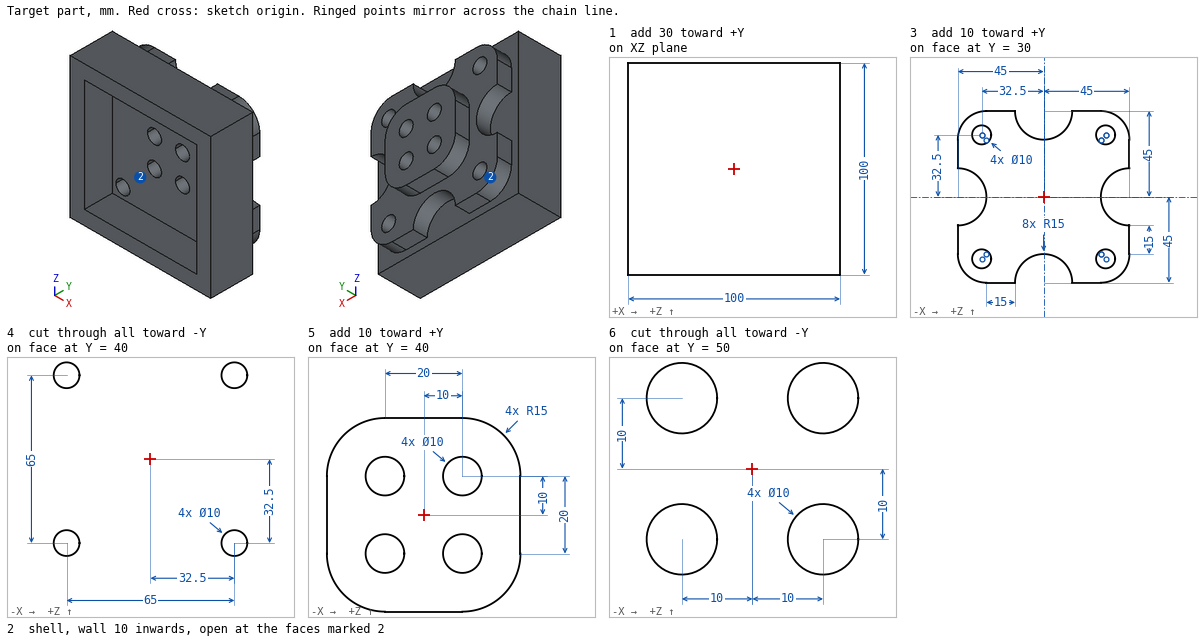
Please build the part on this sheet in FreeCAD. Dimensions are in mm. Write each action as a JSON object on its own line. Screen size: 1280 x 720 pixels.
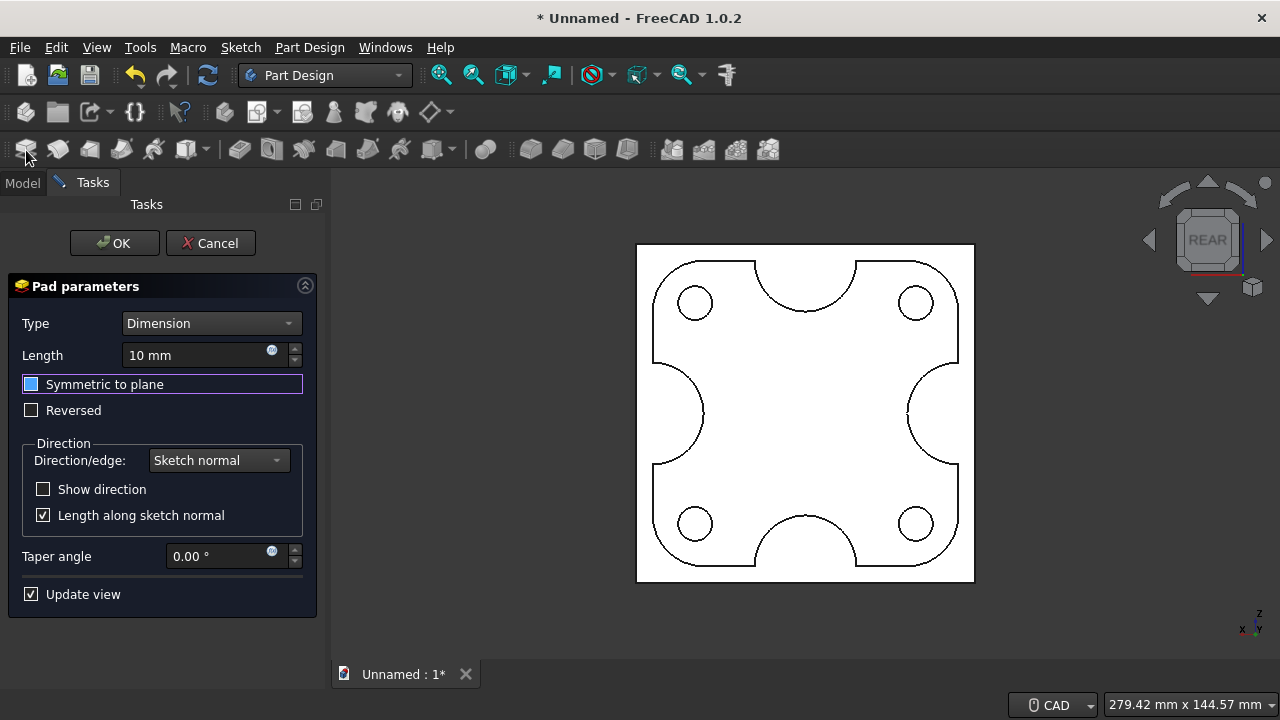
{"action": "left_click", "coordinate": [115, 243]}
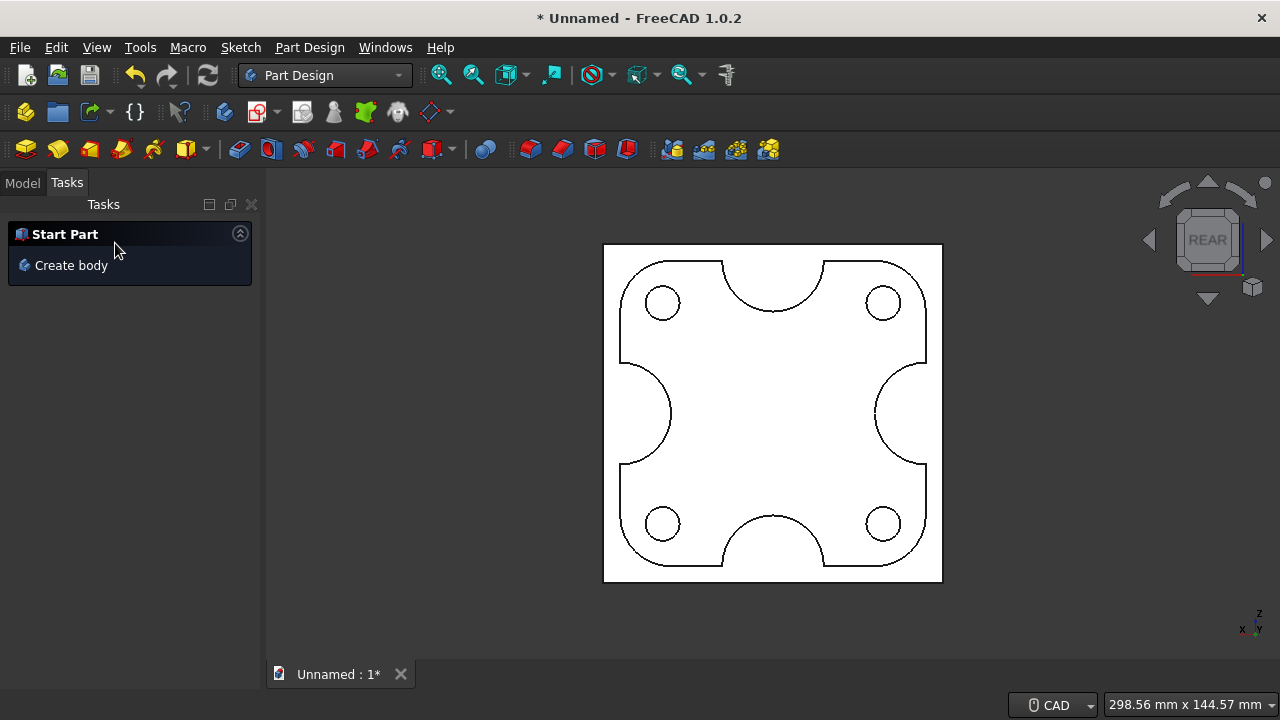
{"action": "left_click", "coordinate": [773, 412]}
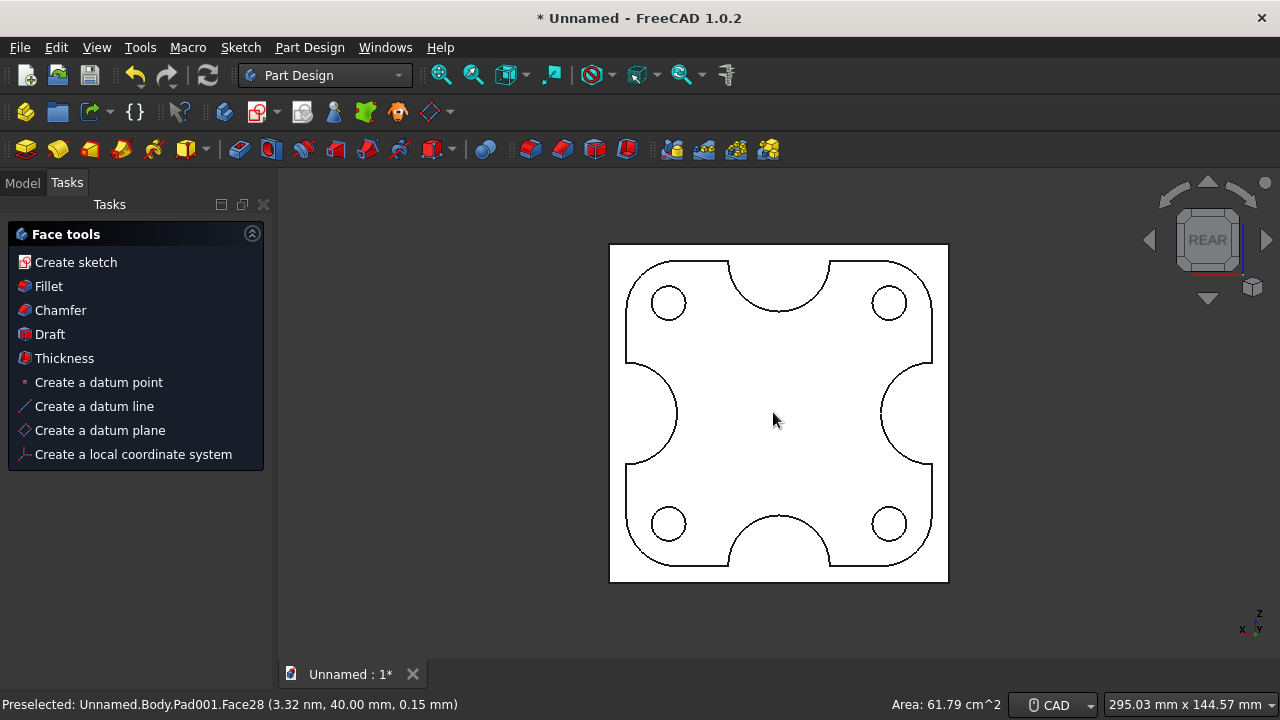
{"action": "left_click", "coordinate": [258, 112]}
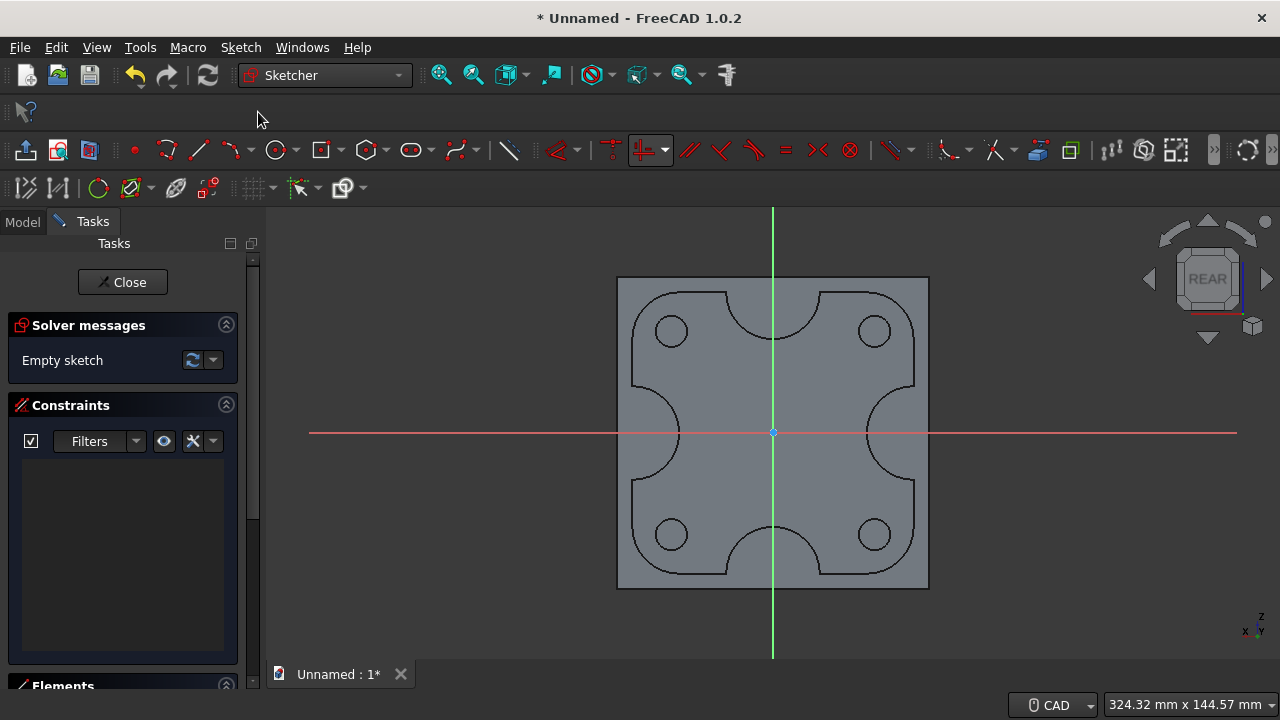
{"action": "left_click", "coordinate": [276, 150]}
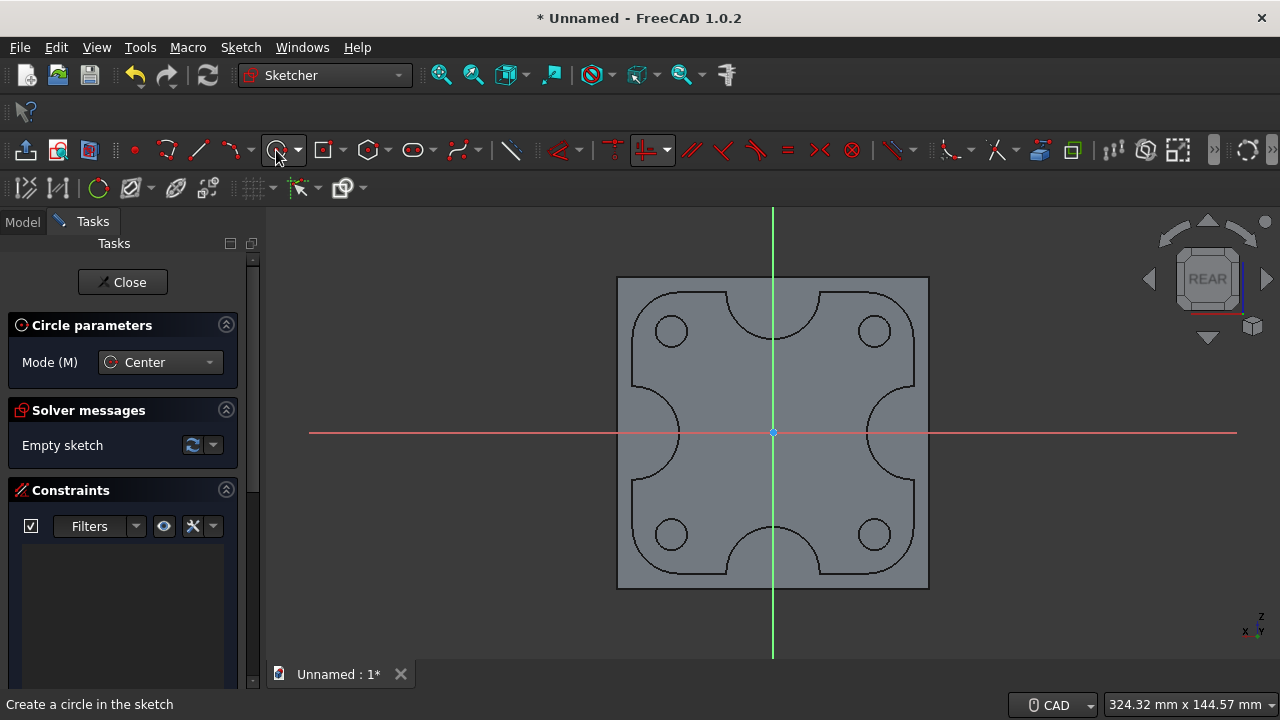
{"action": "scroll", "coordinate": [875, 535], "scroll_direction": "up", "scroll_amount": 2}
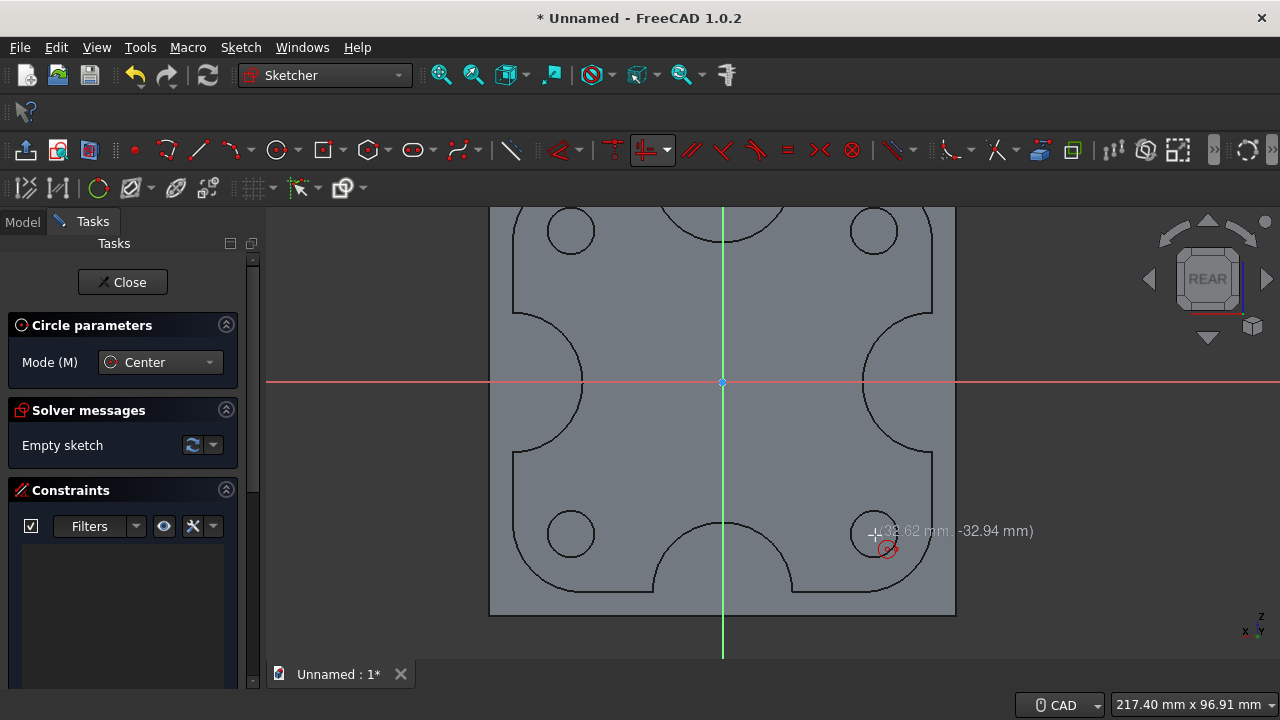
{"action": "left_click", "coordinate": [874, 534]}
{"action": "left_click", "coordinate": [891, 518]}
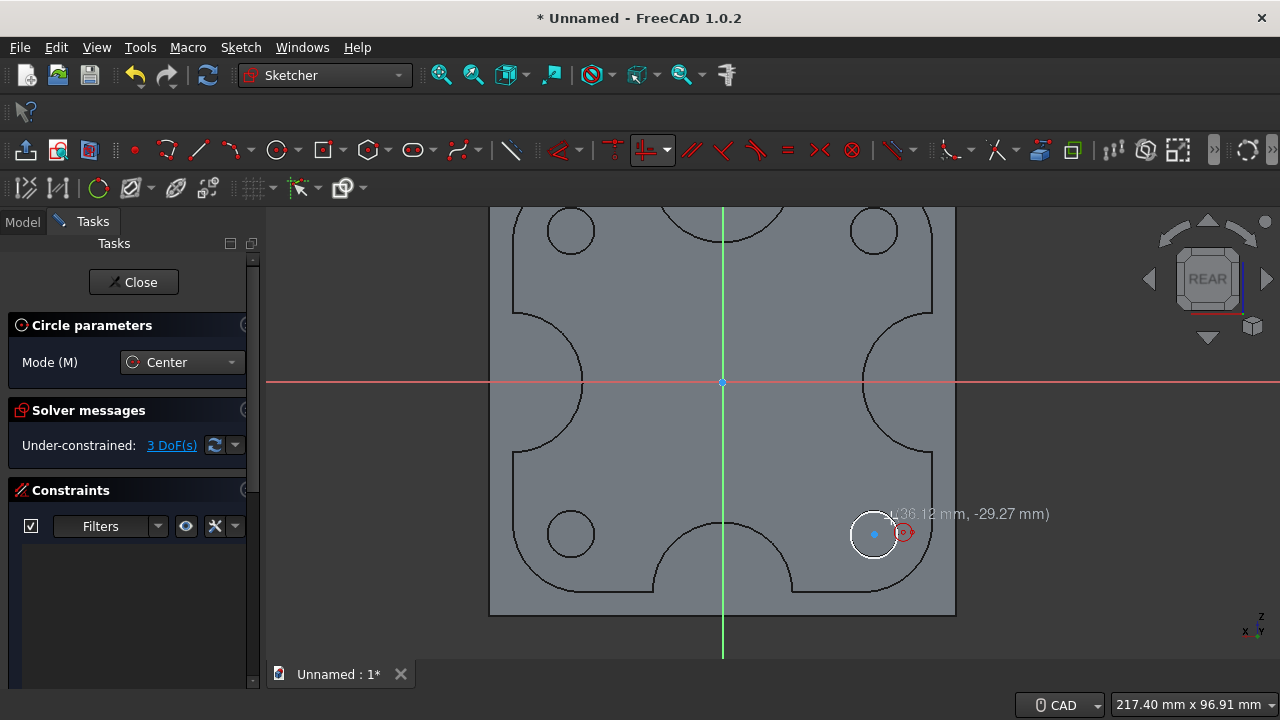
{"action": "left_click", "coordinate": [571, 534]}
{"action": "left_click", "coordinate": [587, 518]}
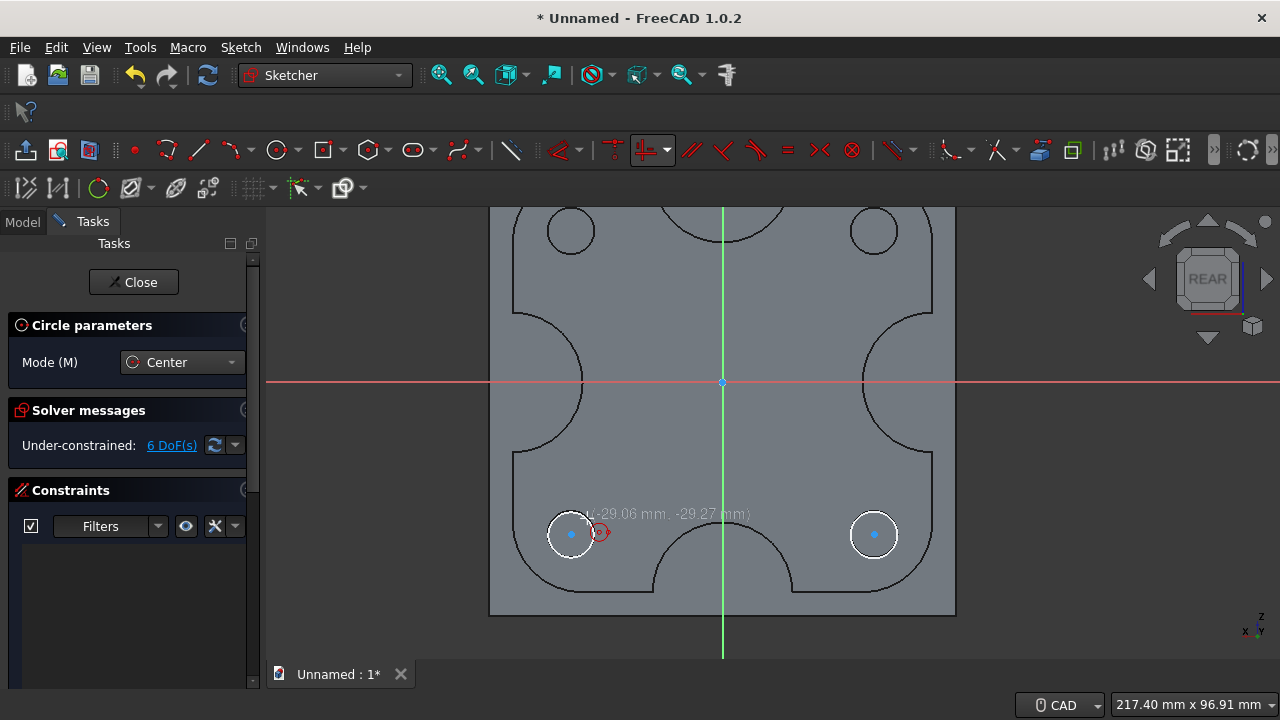
{"action": "scroll", "coordinate": [623, 631], "scroll_direction": "down", "scroll_amount": 1}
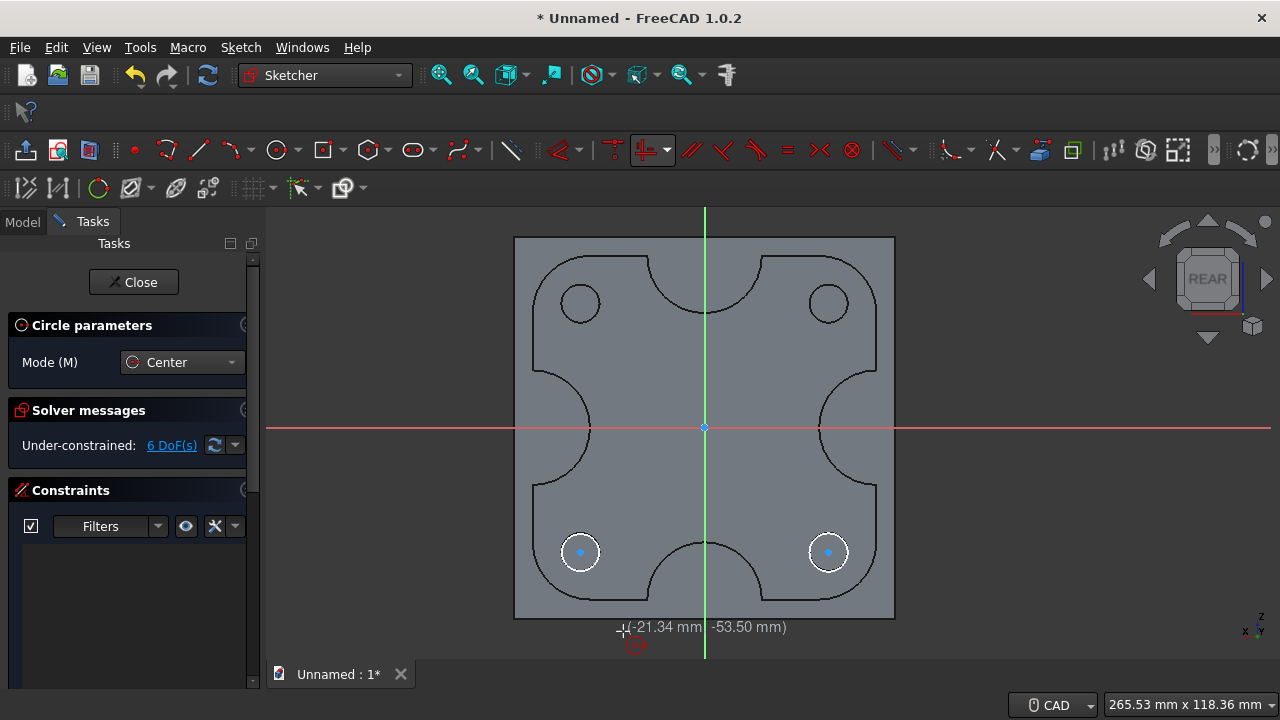
{"action": "left_click", "coordinate": [580, 304]}
{"action": "left_click", "coordinate": [594, 290]}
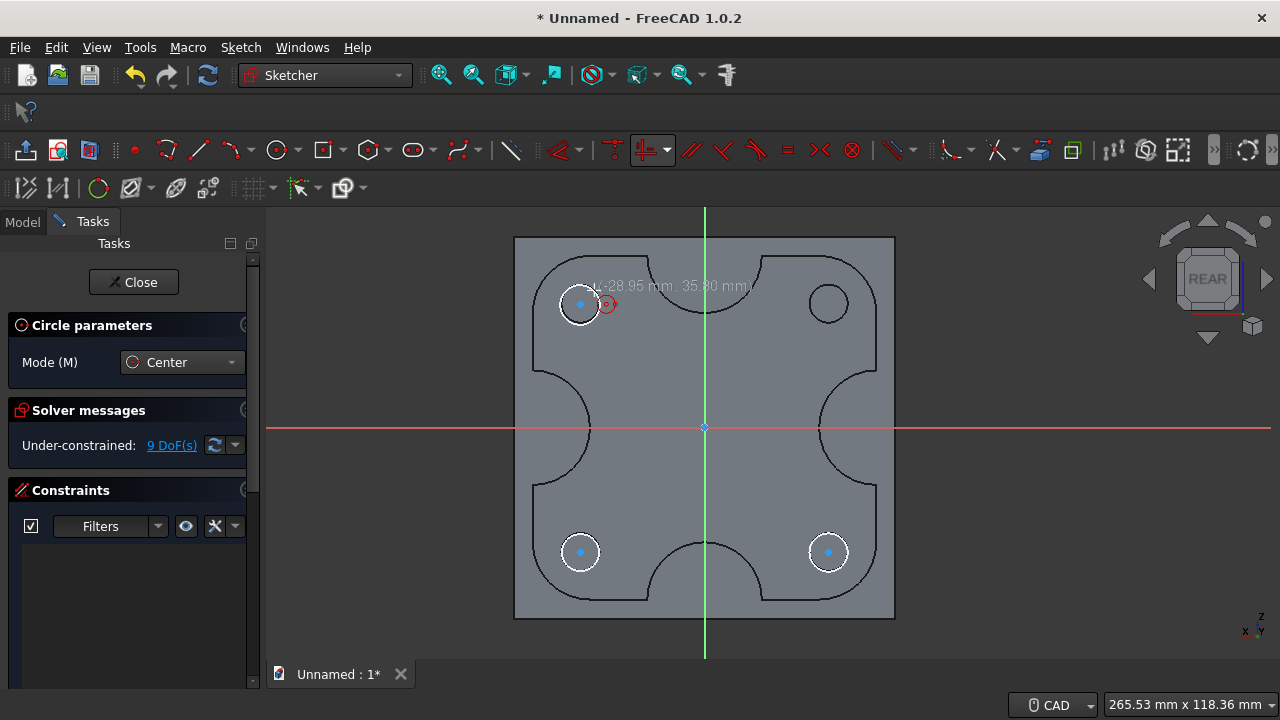
{"action": "left_click", "coordinate": [829, 304]}
{"action": "left_click", "coordinate": [842, 290]}
{"action": "key", "text": "Escape"}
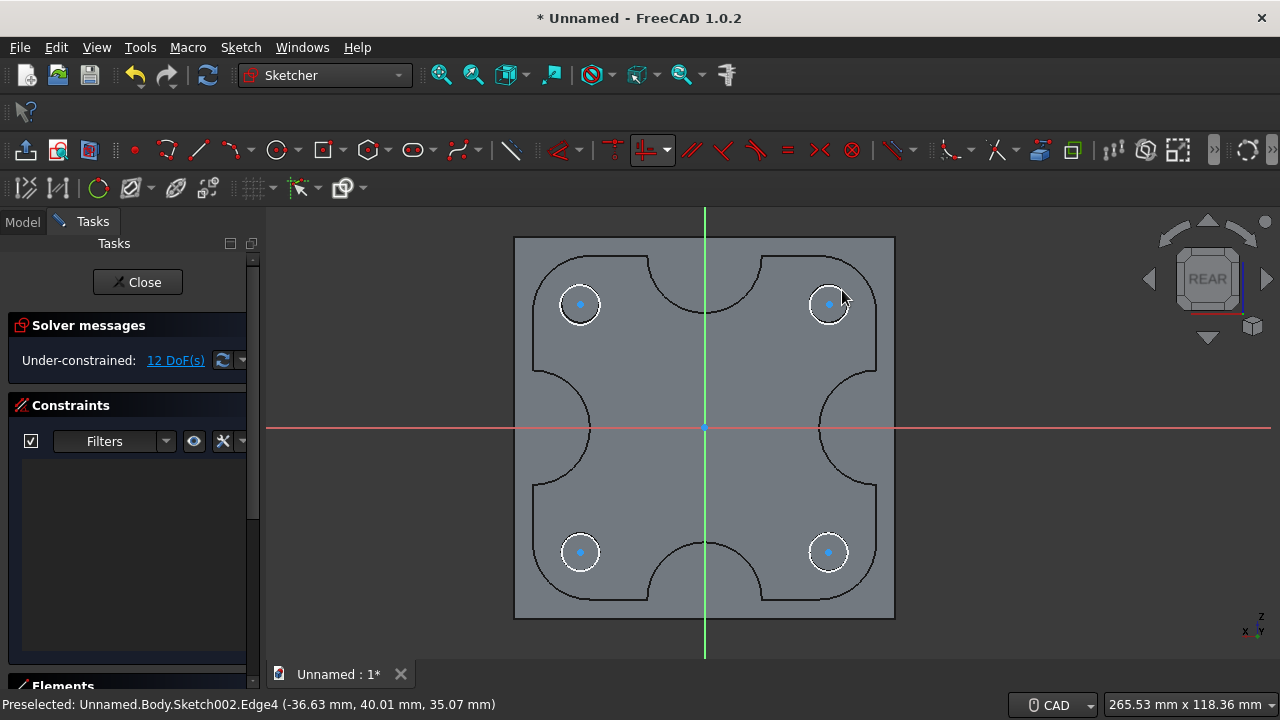
{"action": "left_click", "coordinate": [842, 539]}